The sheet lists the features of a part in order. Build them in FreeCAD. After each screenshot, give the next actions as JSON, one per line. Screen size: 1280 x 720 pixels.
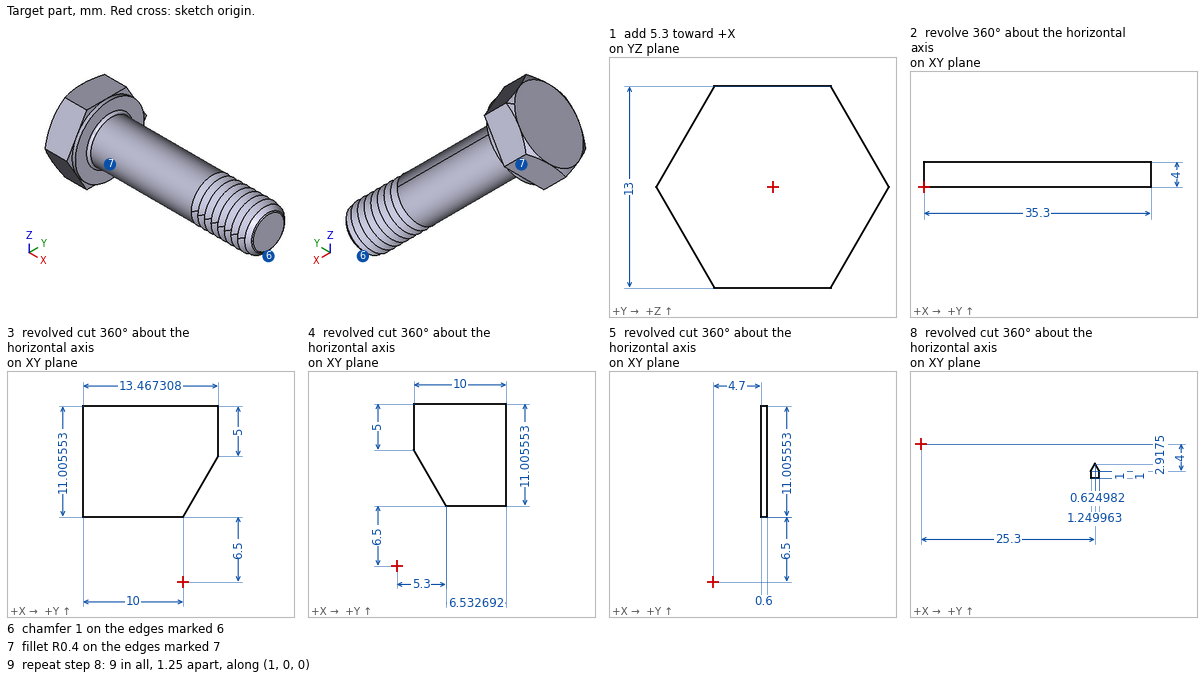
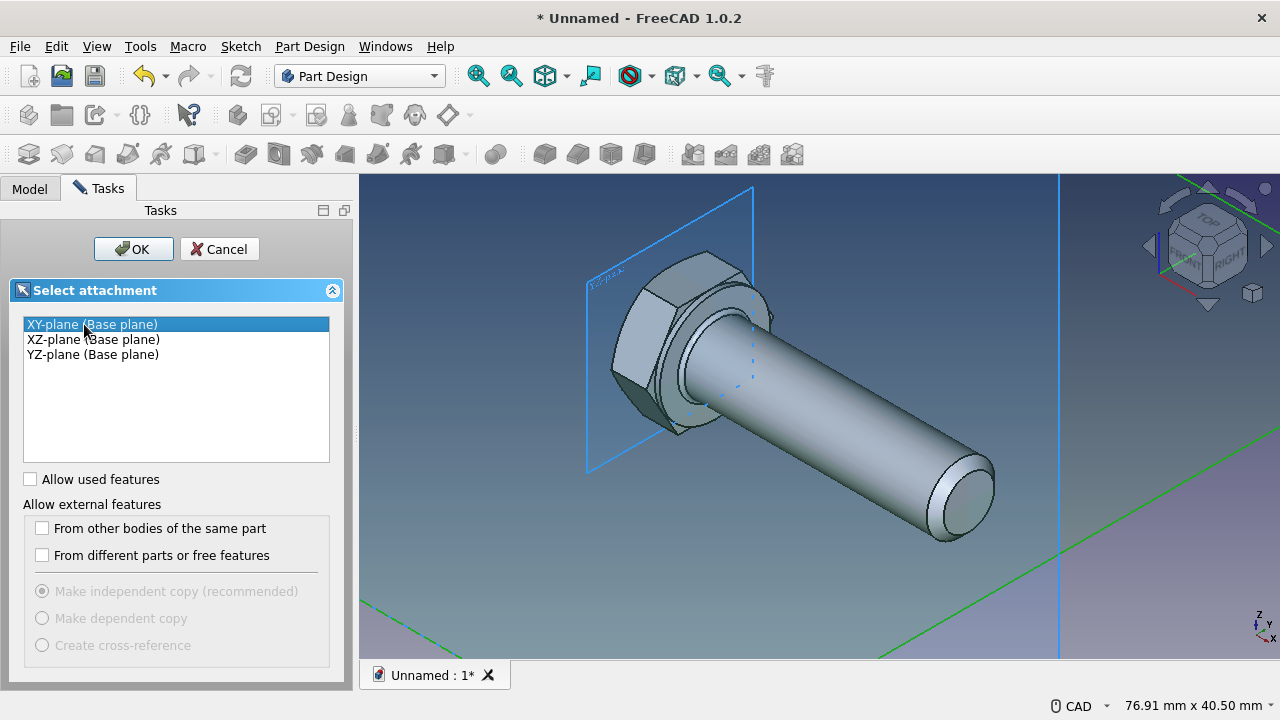
{"action": "left_click", "coordinate": [134, 249]}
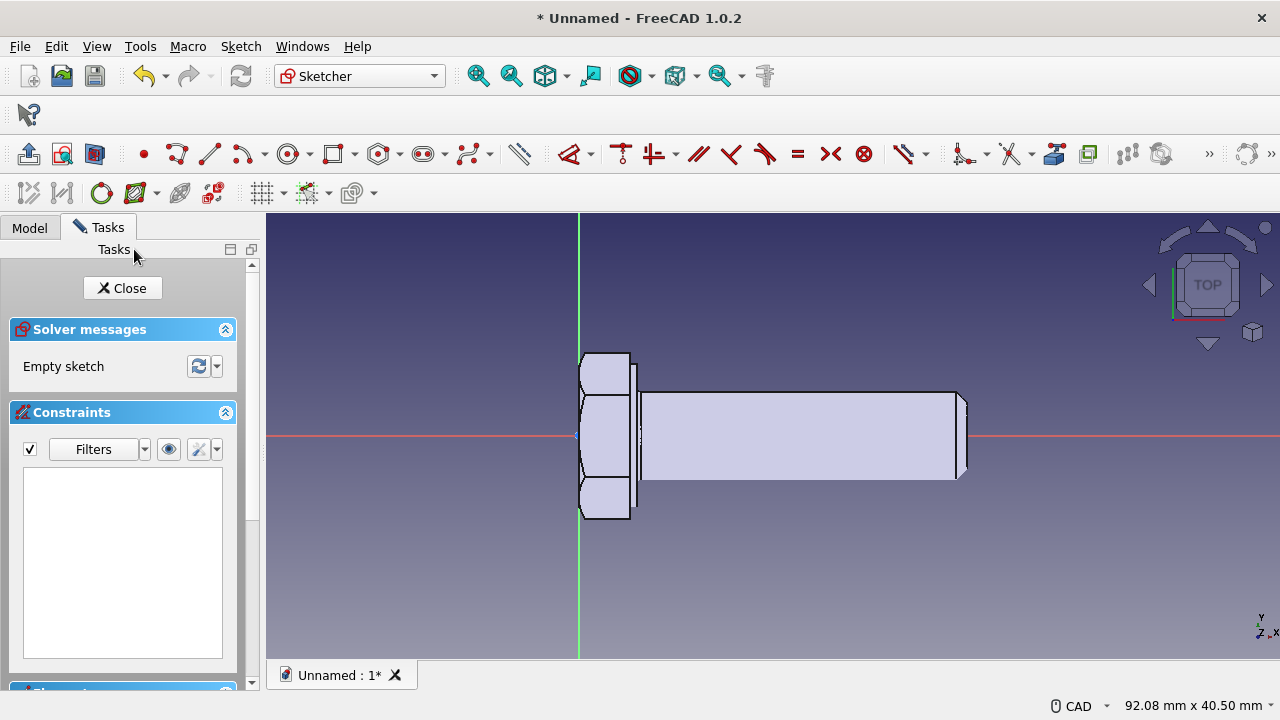
{"action": "left_click", "coordinate": [95, 154]}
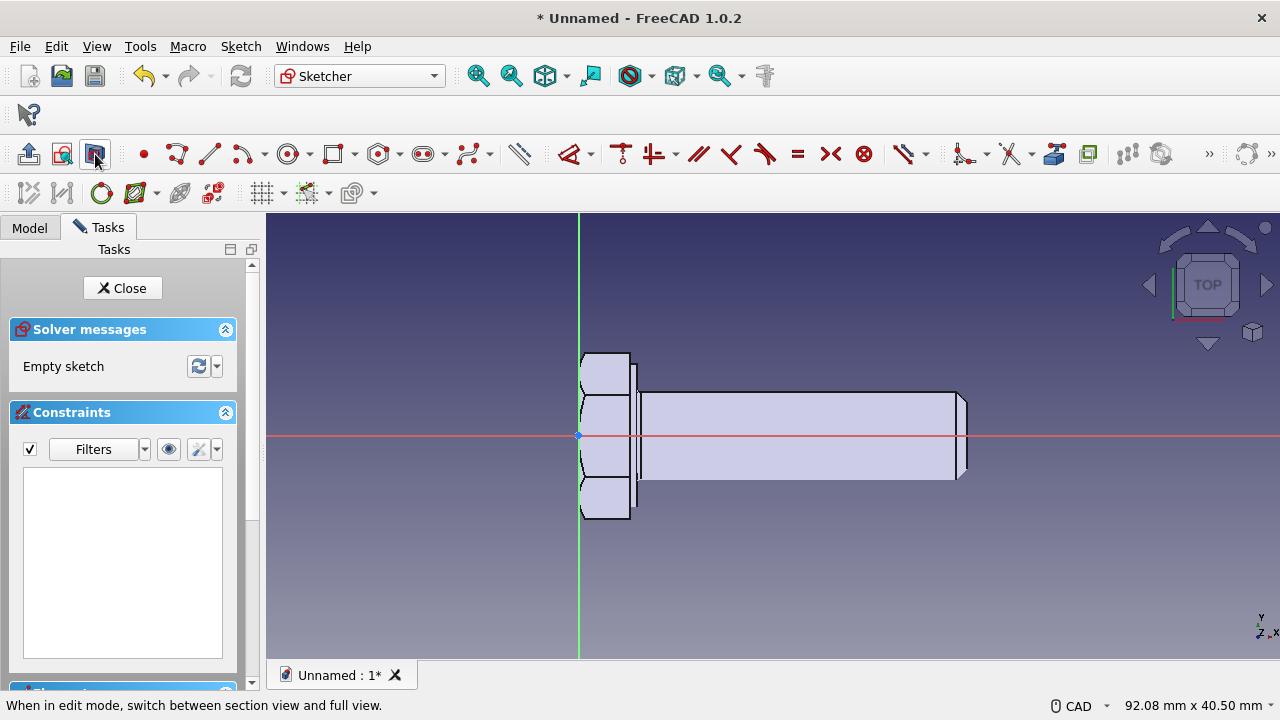
{"action": "scroll", "coordinate": [872, 484], "scroll_direction": "up", "scroll_amount": 12}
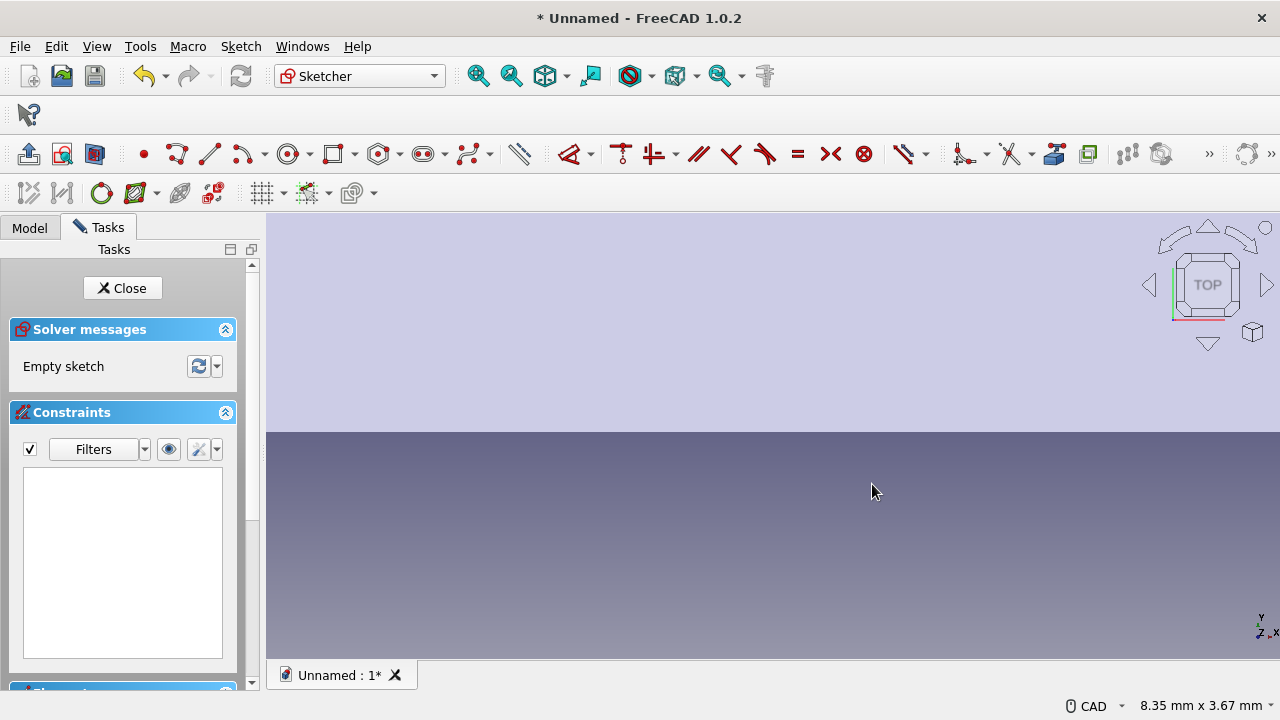
{"action": "left_click", "coordinate": [177, 154]}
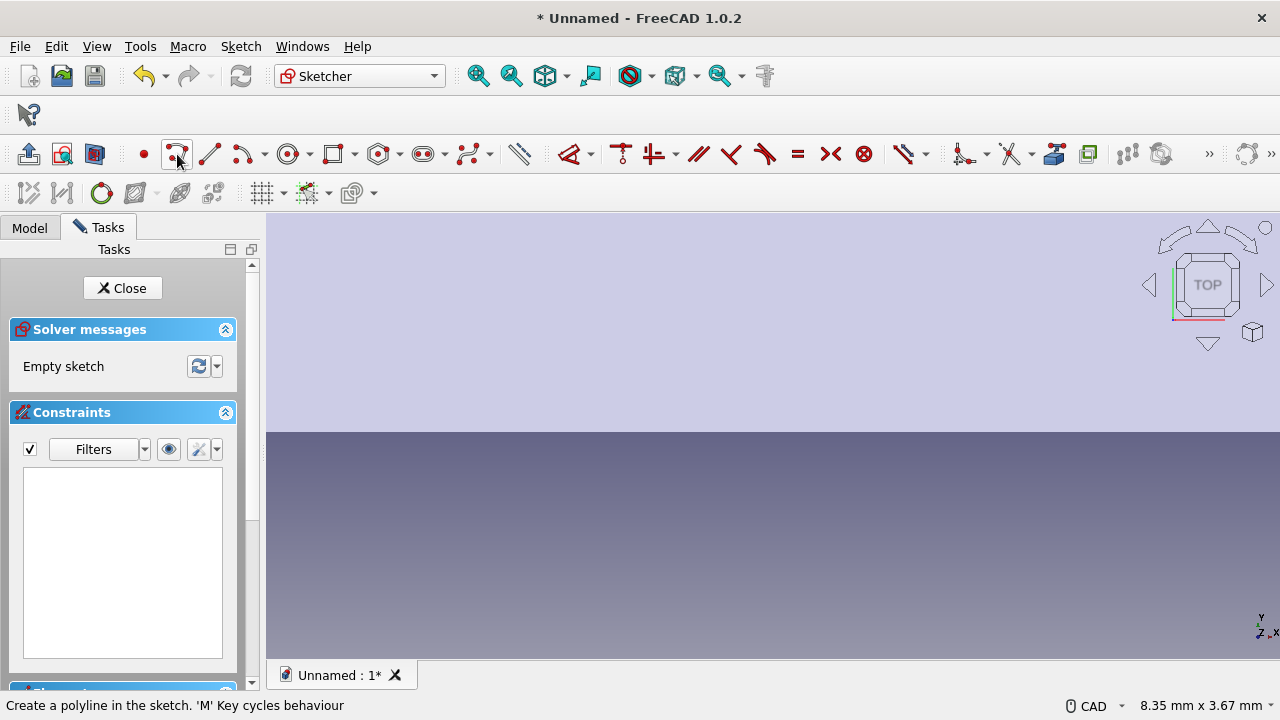
{"action": "left_click", "coordinate": [627, 434]}
{"action": "left_click", "coordinate": [627, 556]}
{"action": "left_click", "coordinate": [779, 556]}
{"action": "left_click", "coordinate": [779, 434]}
{"action": "left_click", "coordinate": [703, 303]}
{"action": "left_click", "coordinate": [627, 435]}
{"action": "key", "text": "Escape"}
{"action": "key", "text": "Escape"}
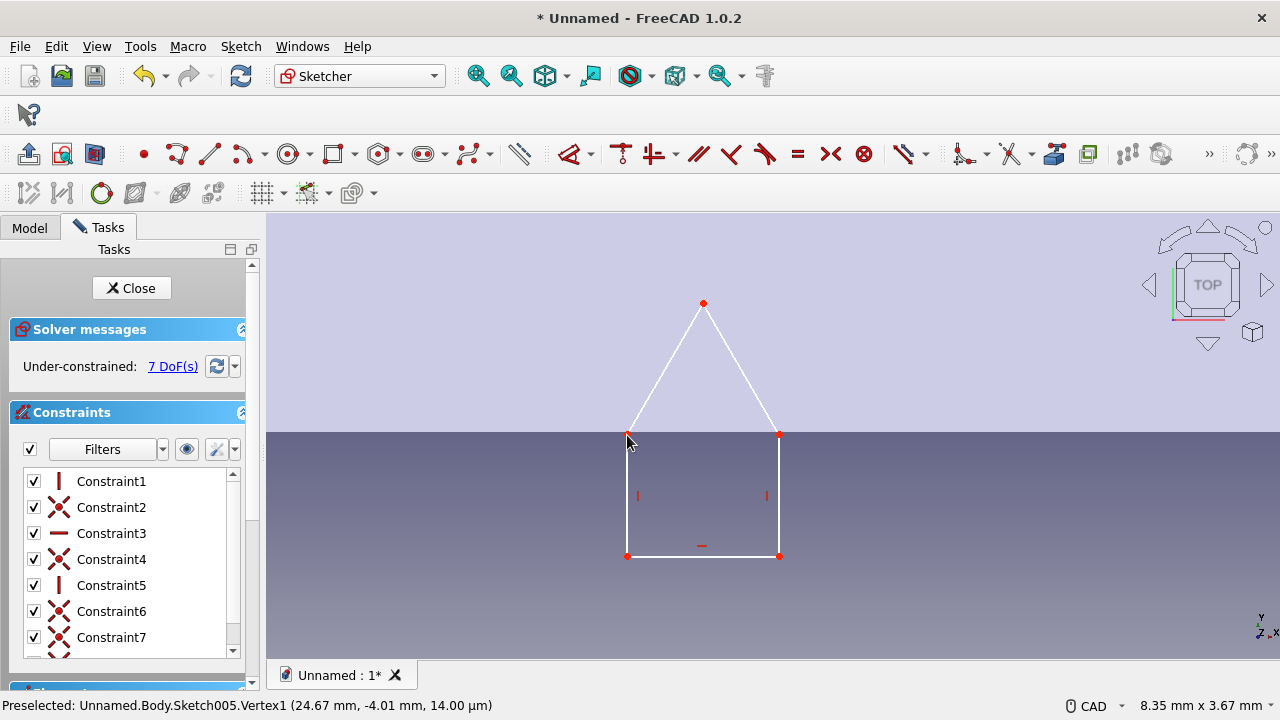
{"action": "key", "text": "d"}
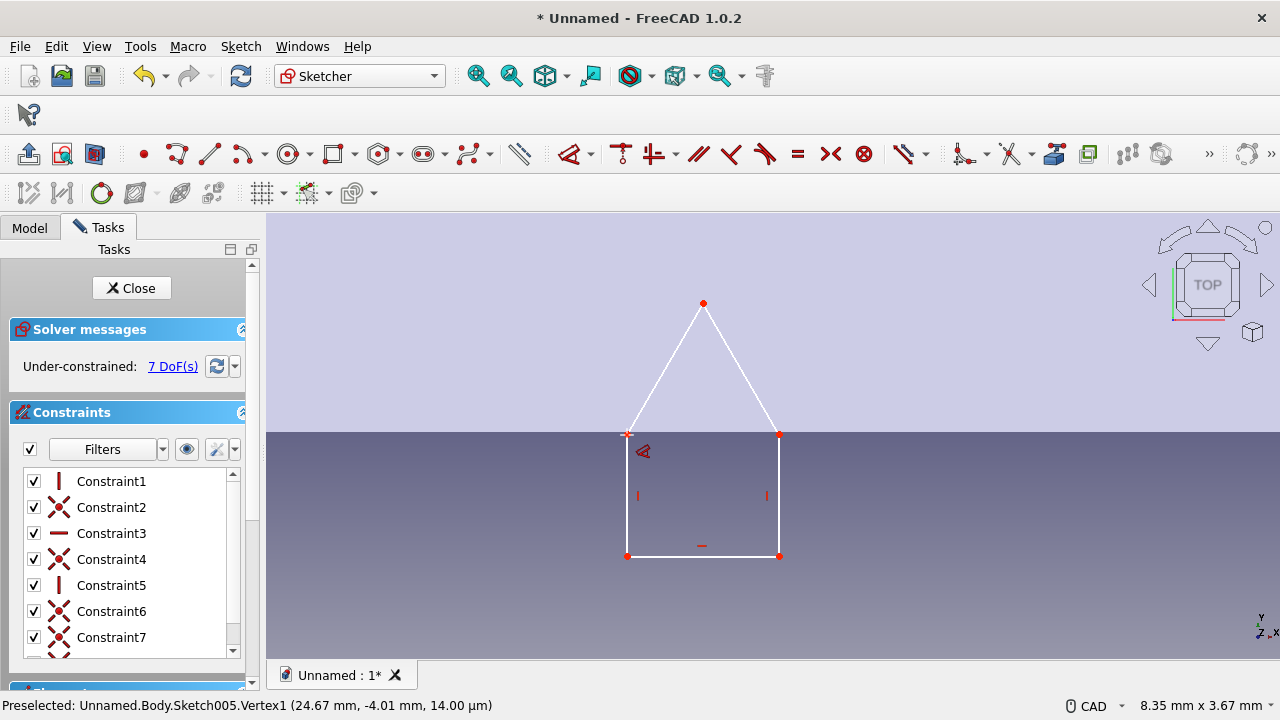
{"action": "left_click", "coordinate": [627, 472]}
{"action": "left_click", "coordinate": [593, 496]}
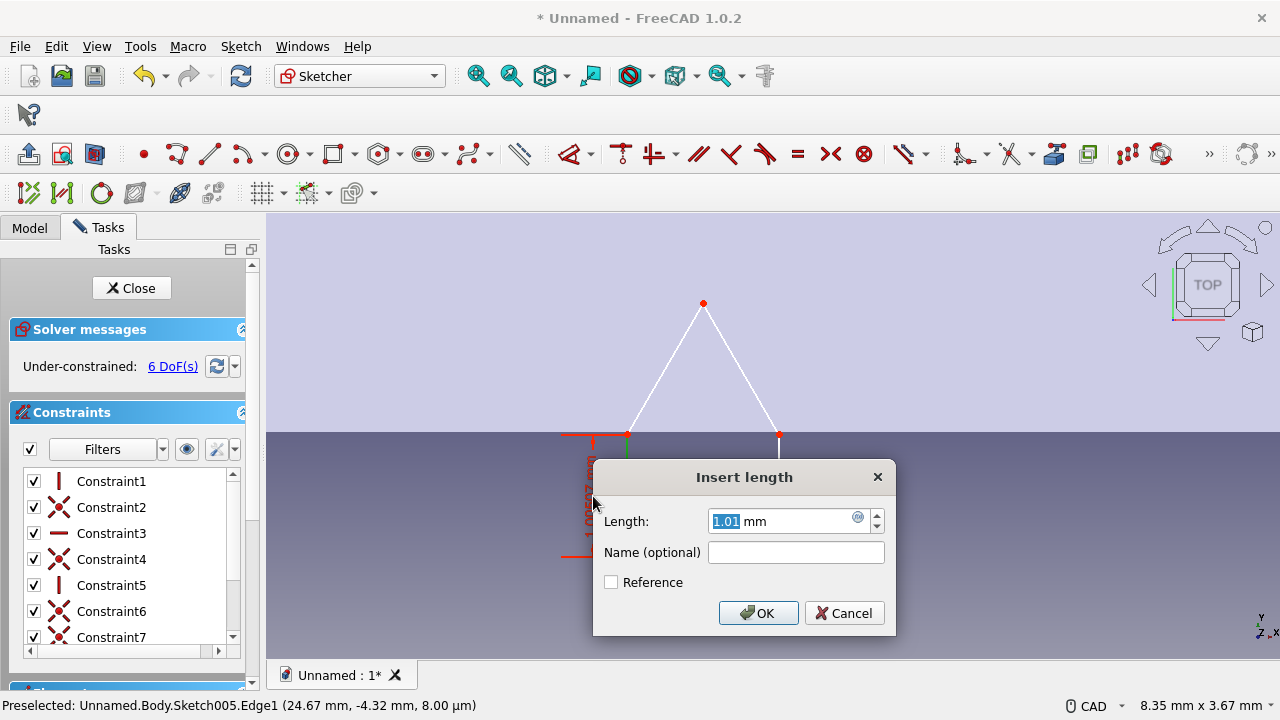
{"action": "type", "text": "1"}
{"action": "key", "text": "Return"}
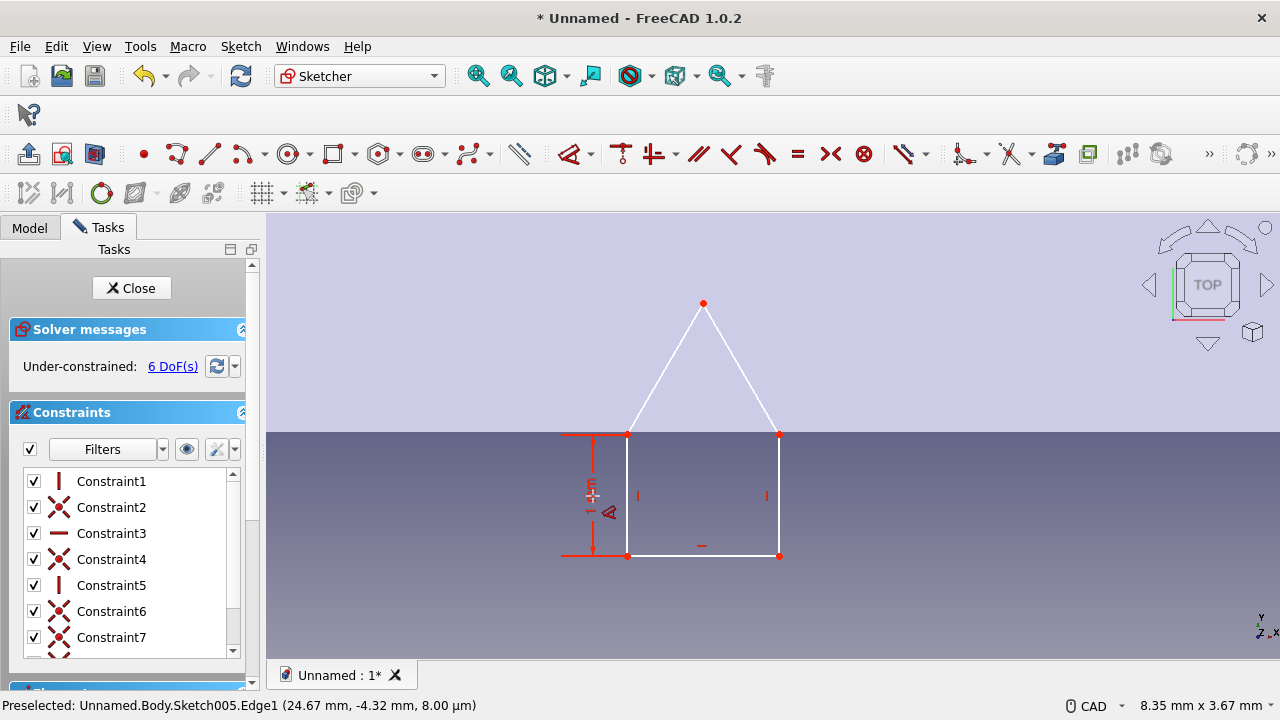
{"action": "left_click", "coordinate": [779, 520]}
{"action": "left_click", "coordinate": [813, 496]}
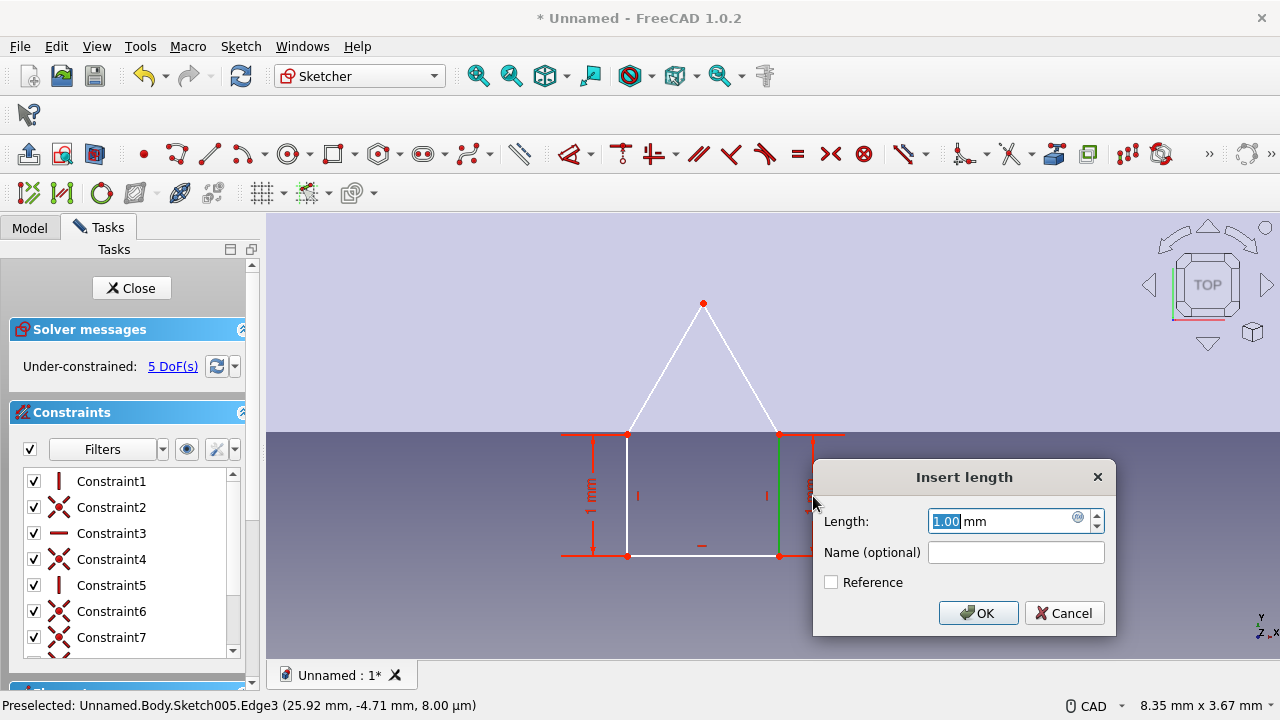
{"action": "type", "text": "1"}
{"action": "key", "text": "Return"}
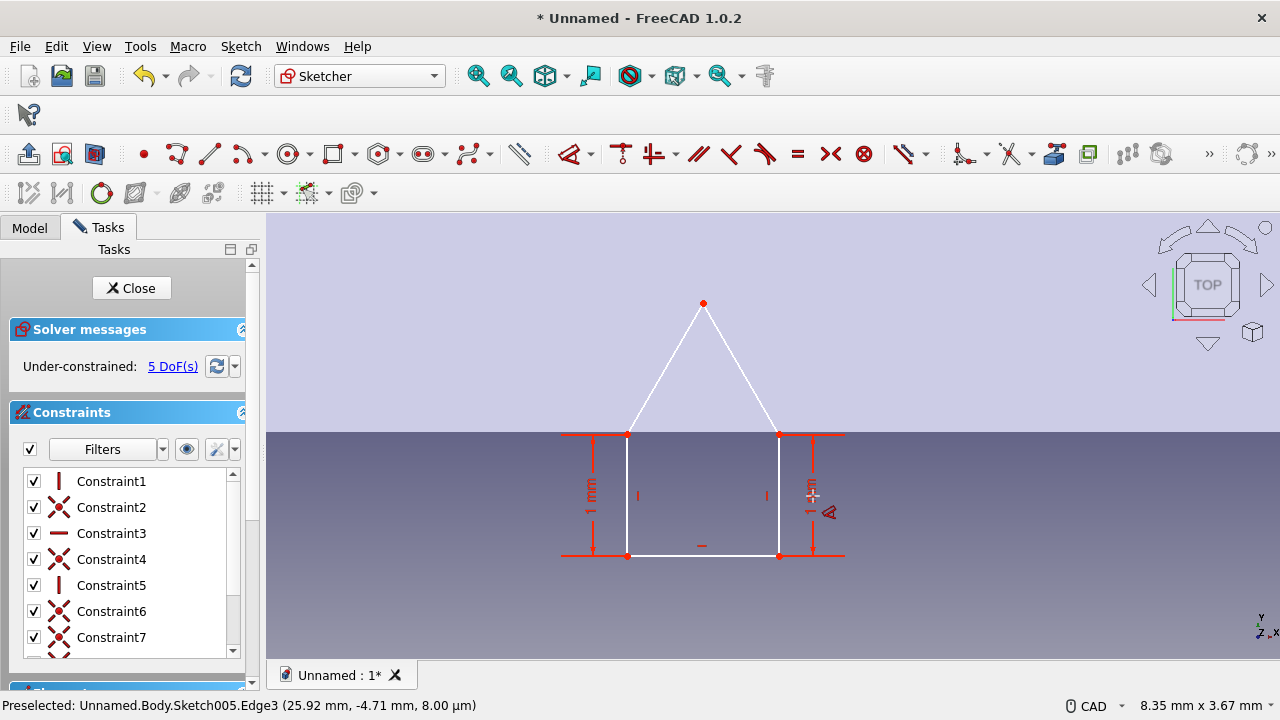
{"action": "left_click", "coordinate": [627, 435]}
{"action": "left_click", "coordinate": [661, 338]}